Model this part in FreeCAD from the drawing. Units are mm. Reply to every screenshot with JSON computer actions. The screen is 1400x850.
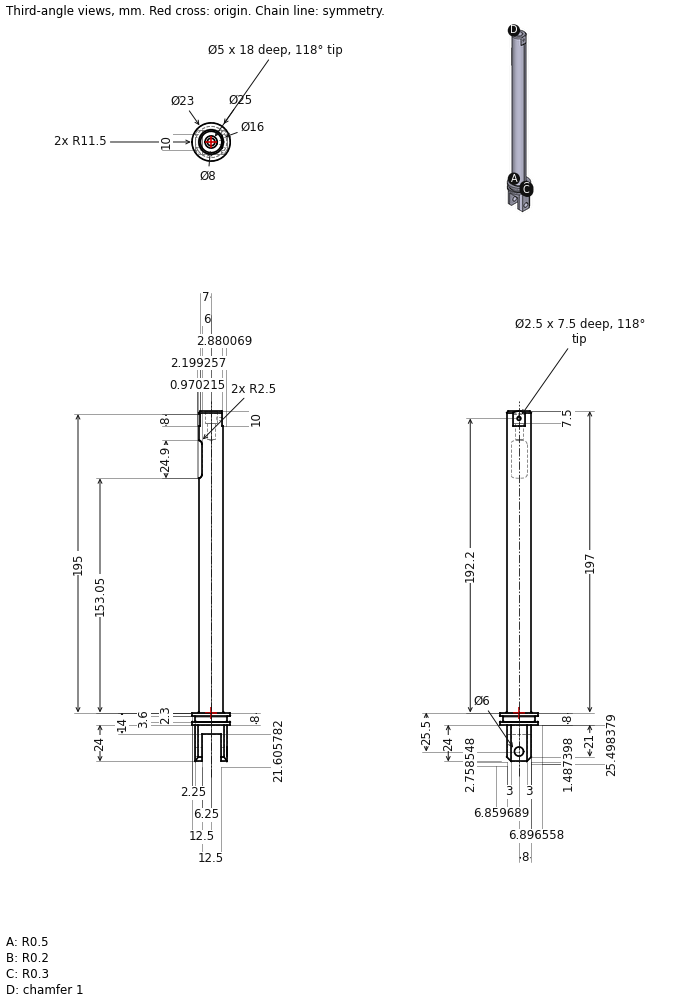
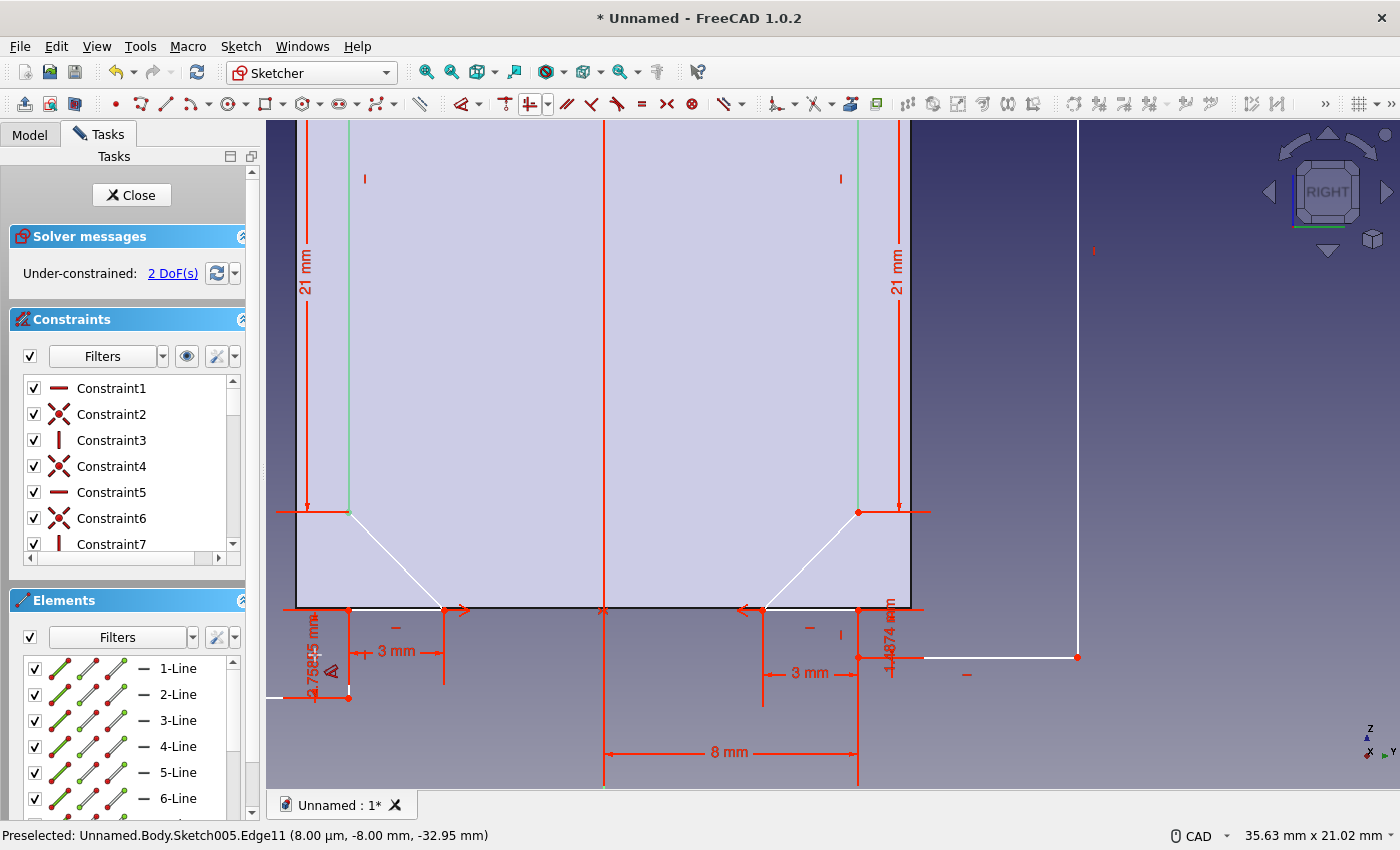
{"action": "left_click", "coordinate": [305, 698]}
{"action": "left_click", "coordinate": [321, 732]}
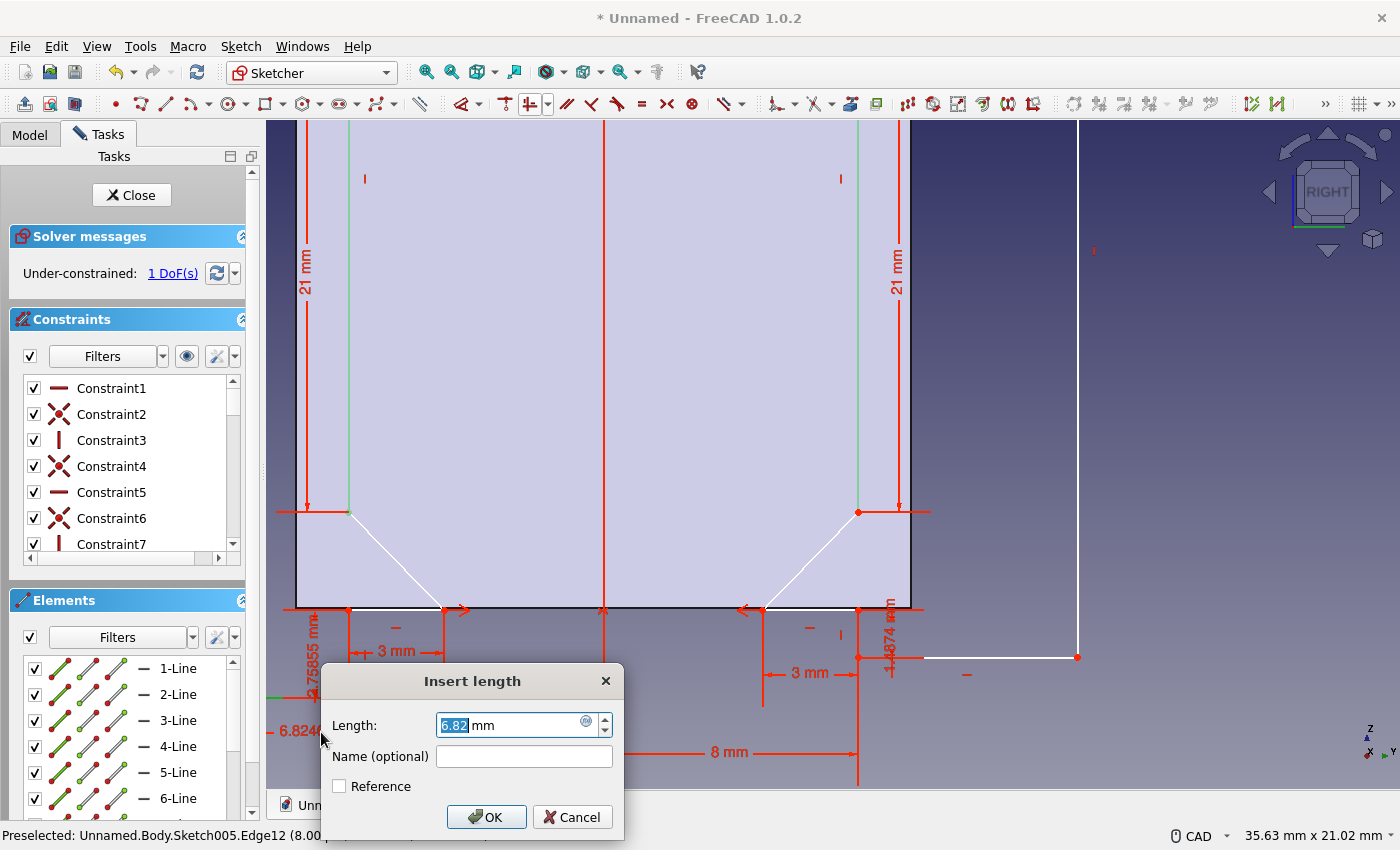
{"action": "type", "text": "6.859689"}
{"action": "key", "text": "Return"}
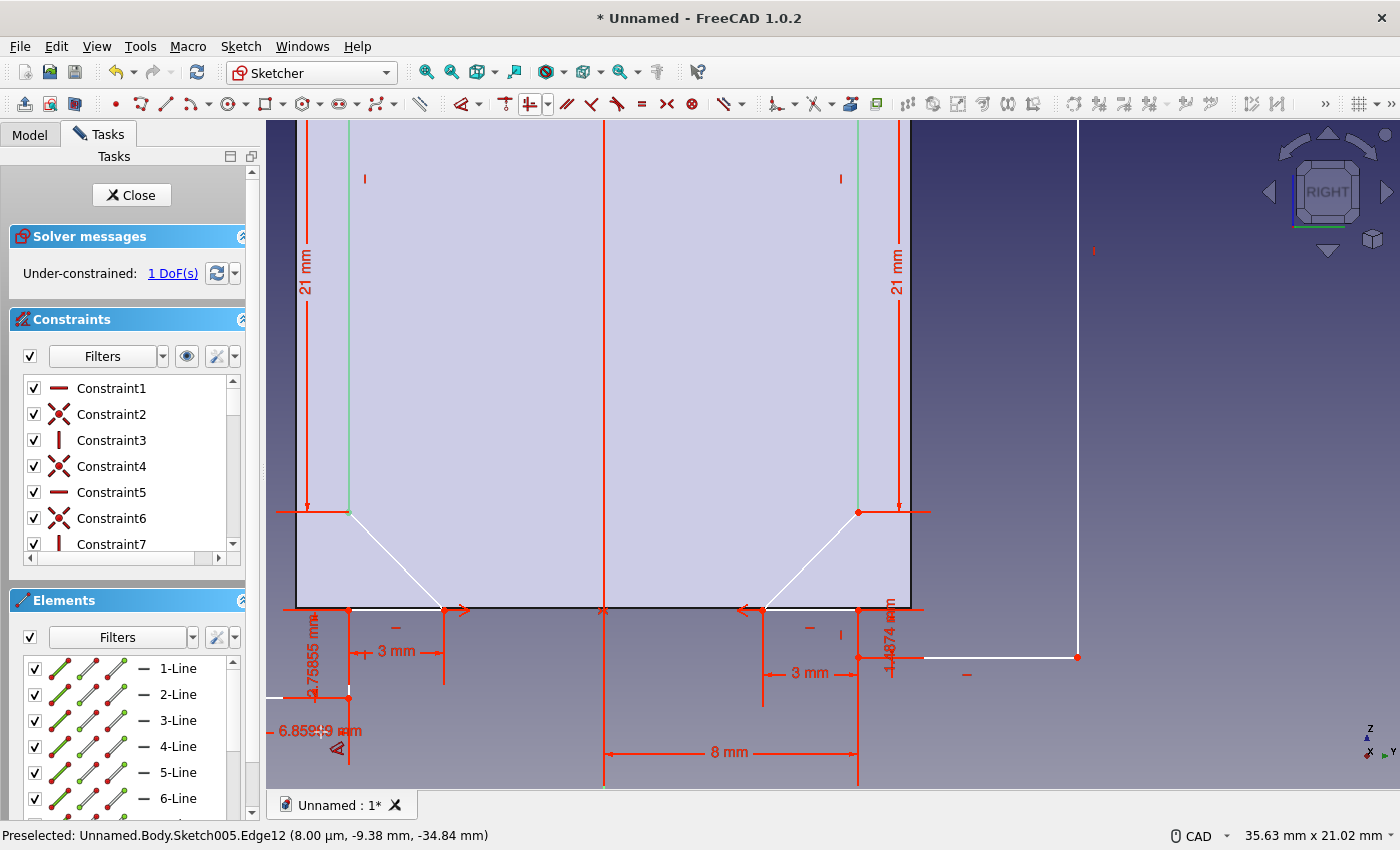
{"action": "left_click", "coordinate": [1078, 414]}
{"action": "left_click", "coordinate": [1112, 403]}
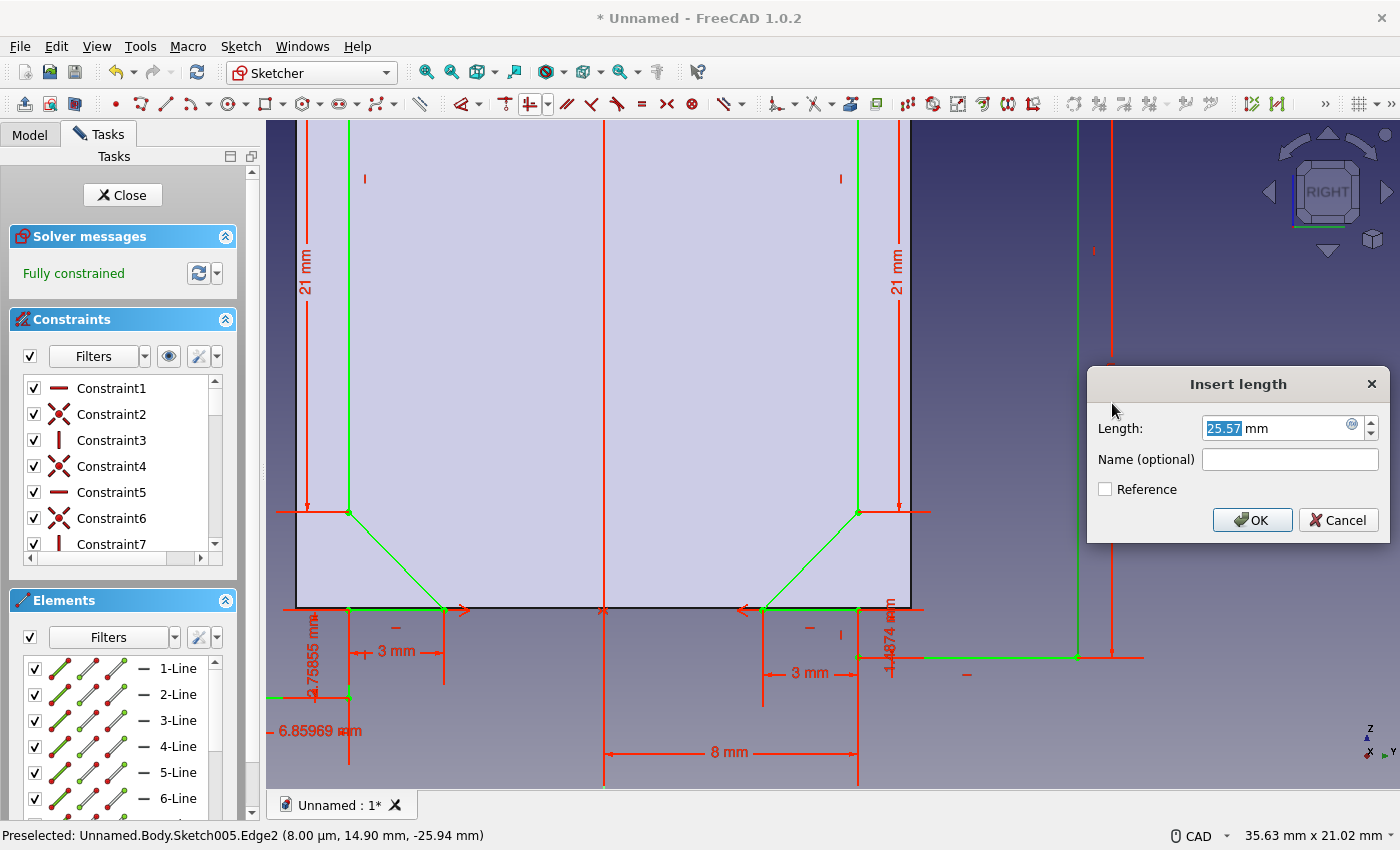
{"action": "type", "text": "25.498379"}
{"action": "key", "text": "Return"}
{"action": "key", "text": "Escape"}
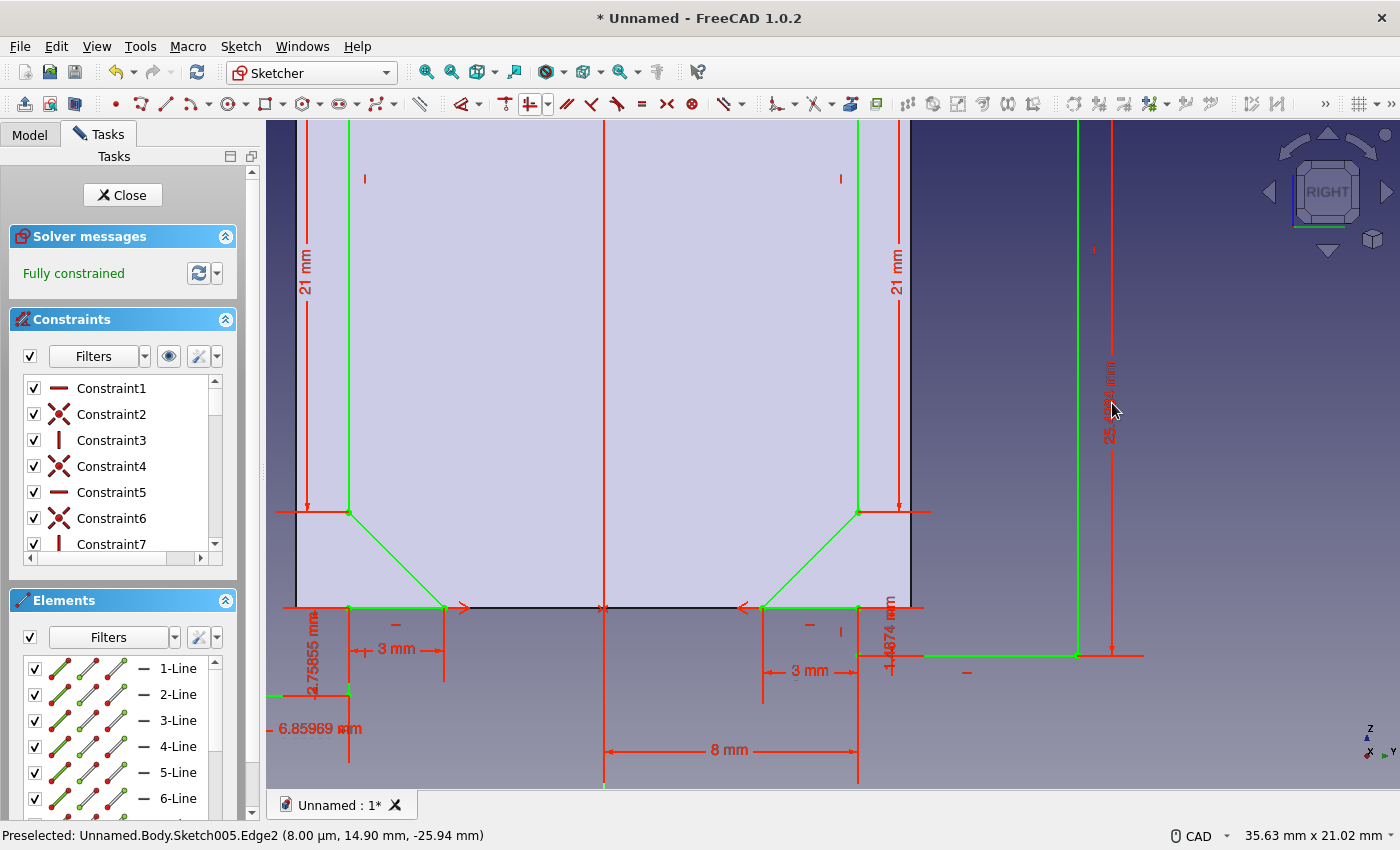
{"action": "left_click", "coordinate": [123, 195]}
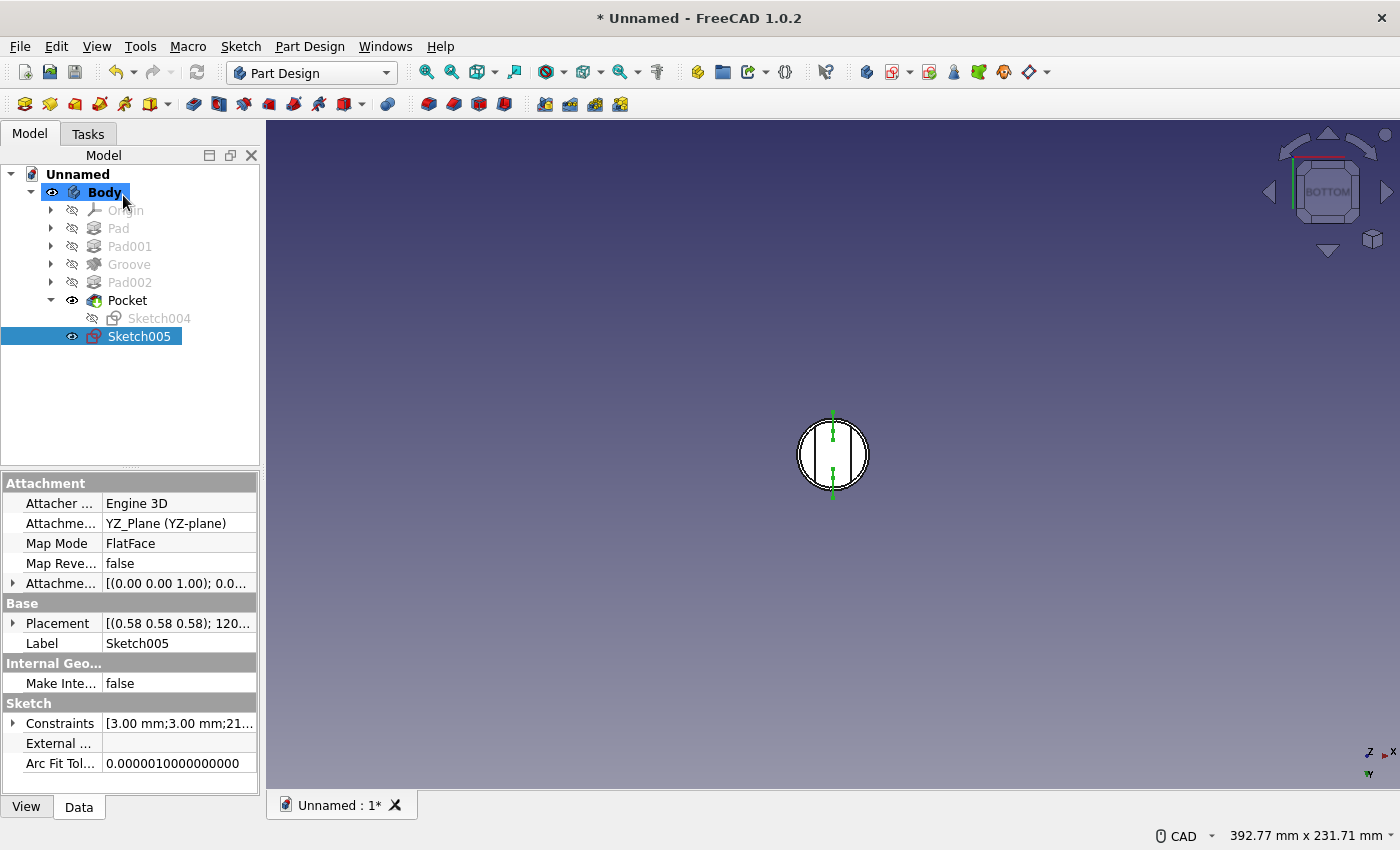
{"action": "left_click", "coordinate": [194, 104]}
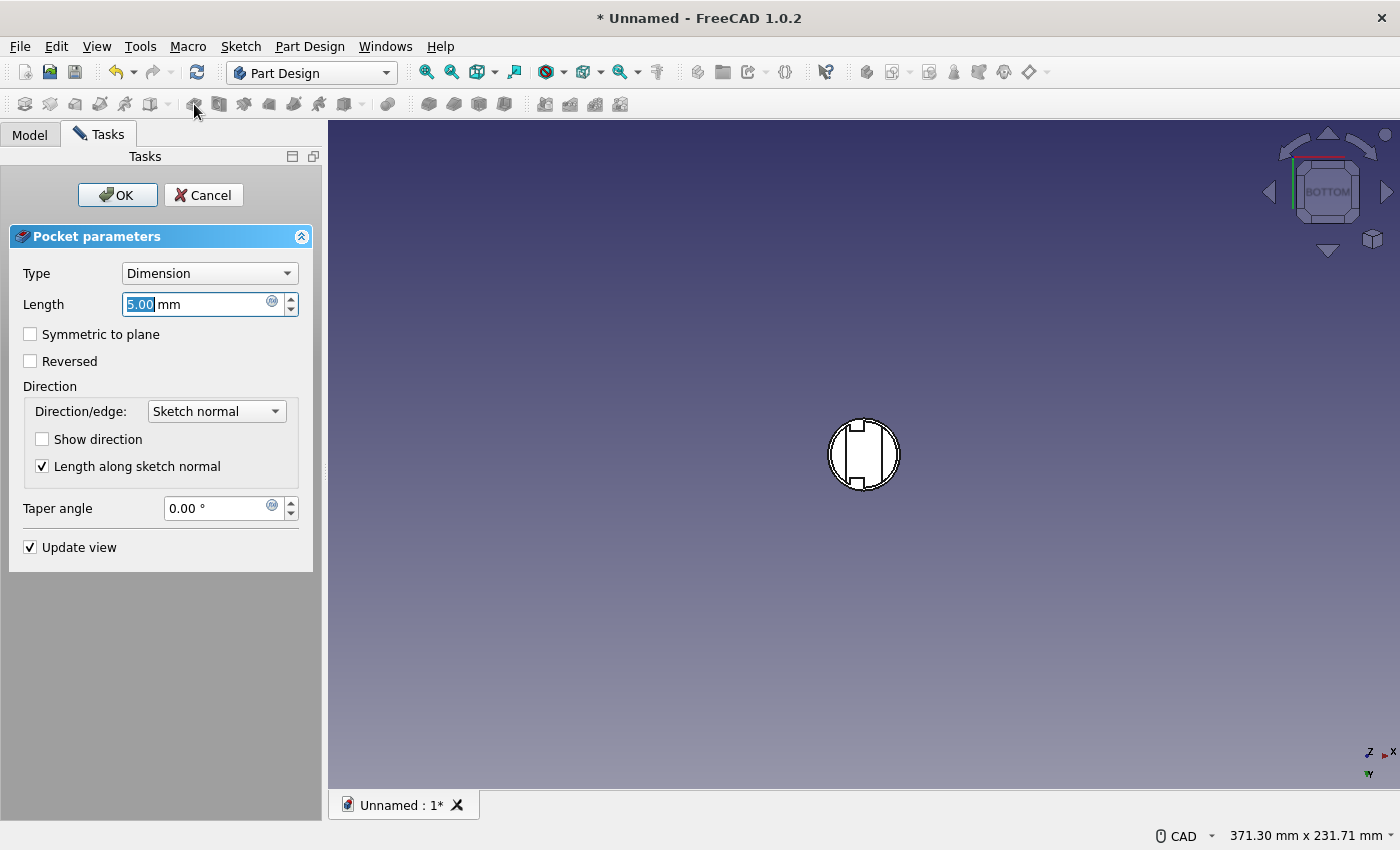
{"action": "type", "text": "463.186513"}
{"action": "key", "text": "Tab"}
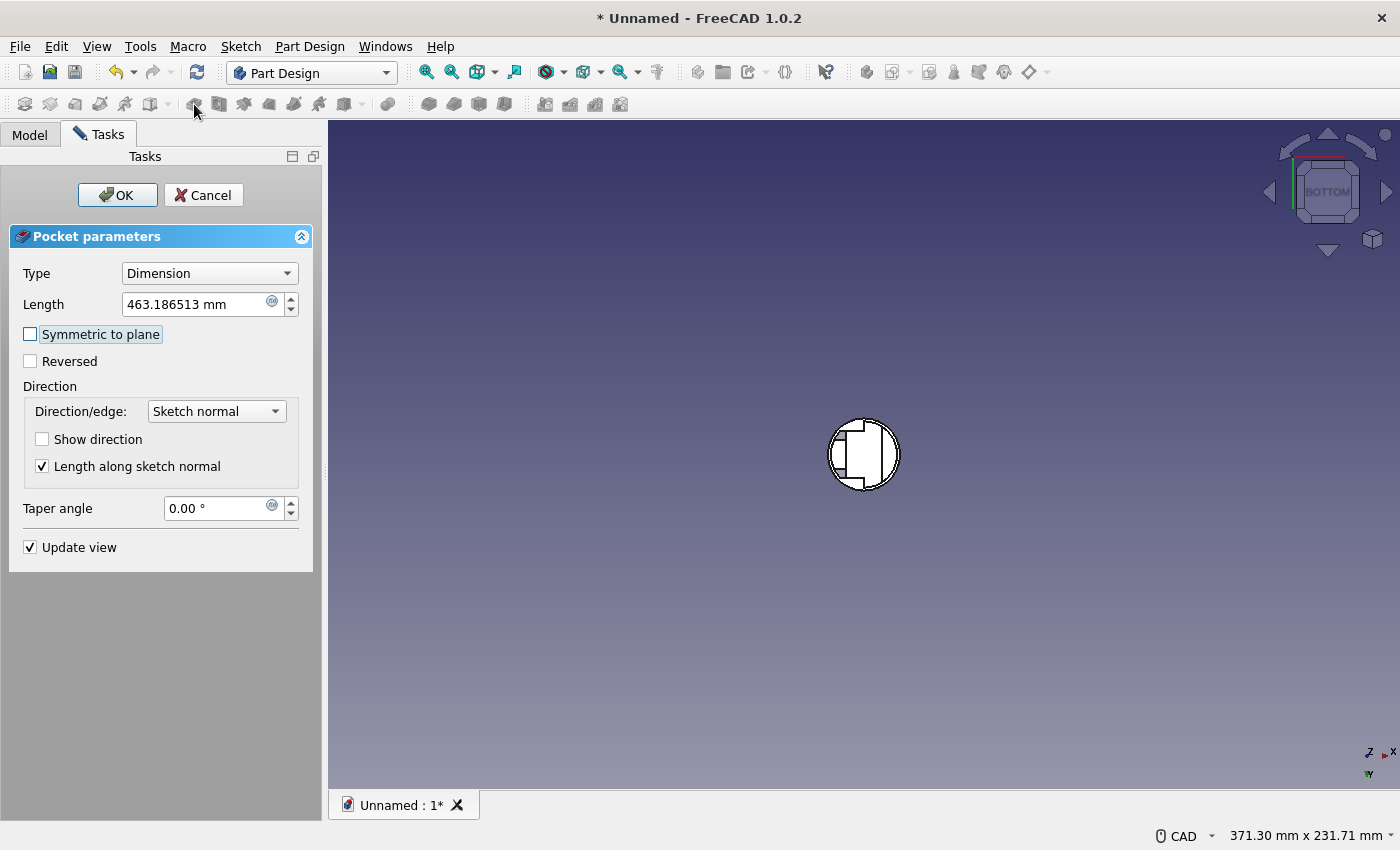
{"action": "left_click", "coordinate": [31, 334]}